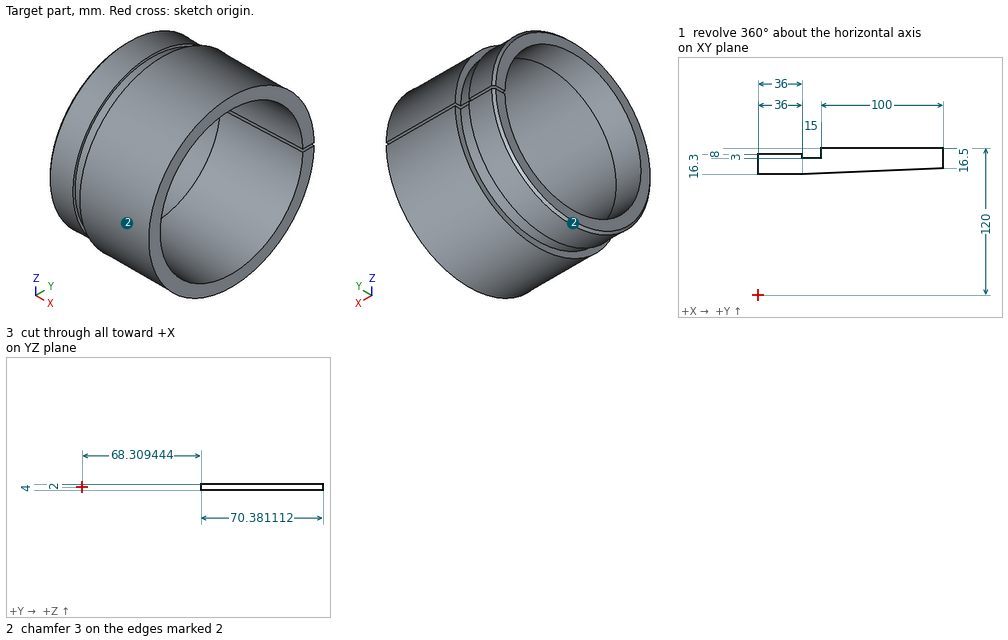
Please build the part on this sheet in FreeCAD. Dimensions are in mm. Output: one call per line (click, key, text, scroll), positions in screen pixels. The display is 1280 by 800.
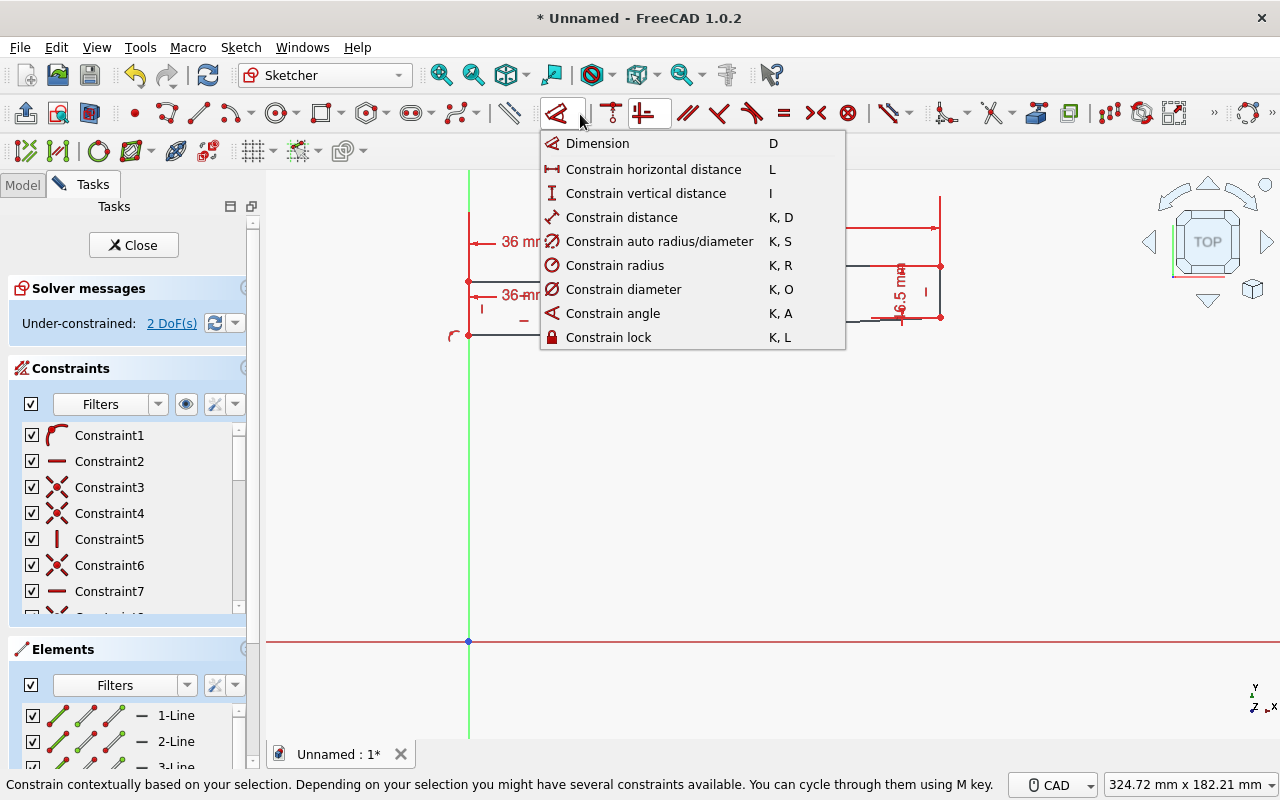
click(693, 193)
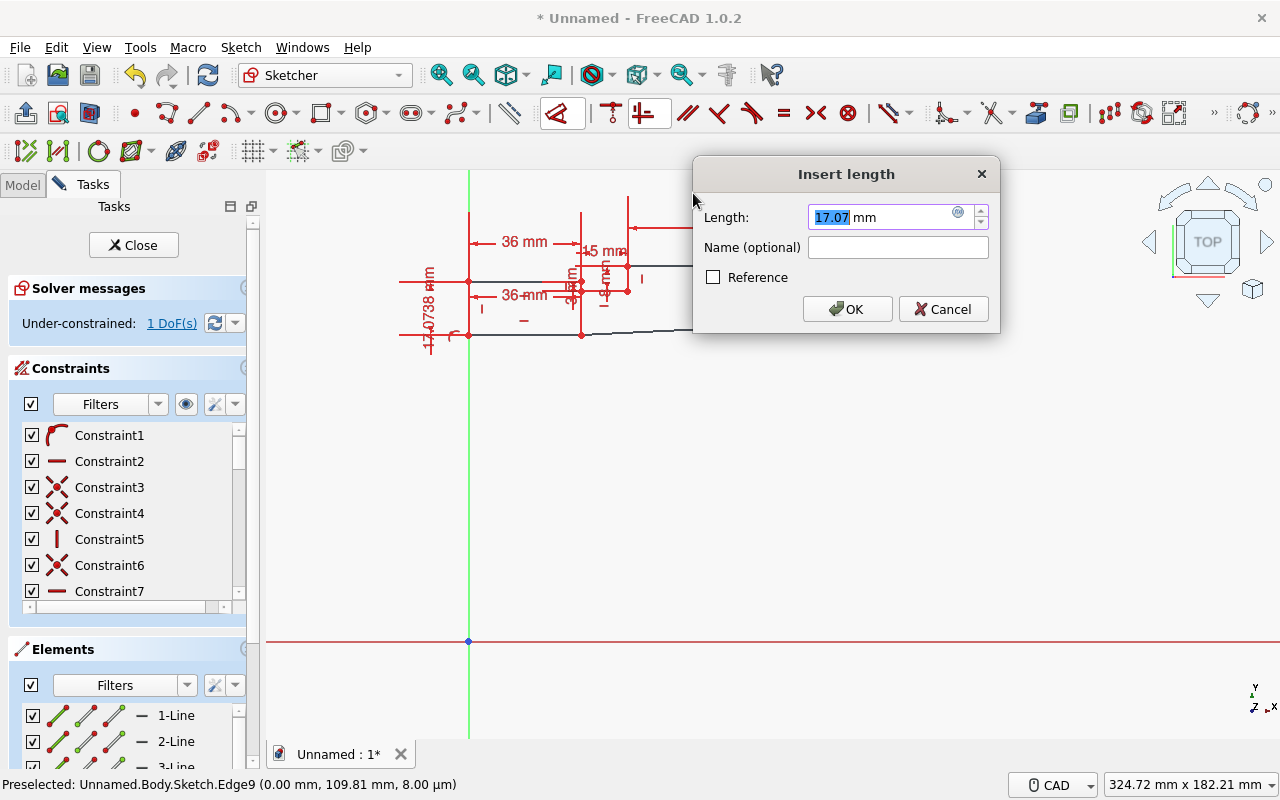
text(16.3)
key(Return)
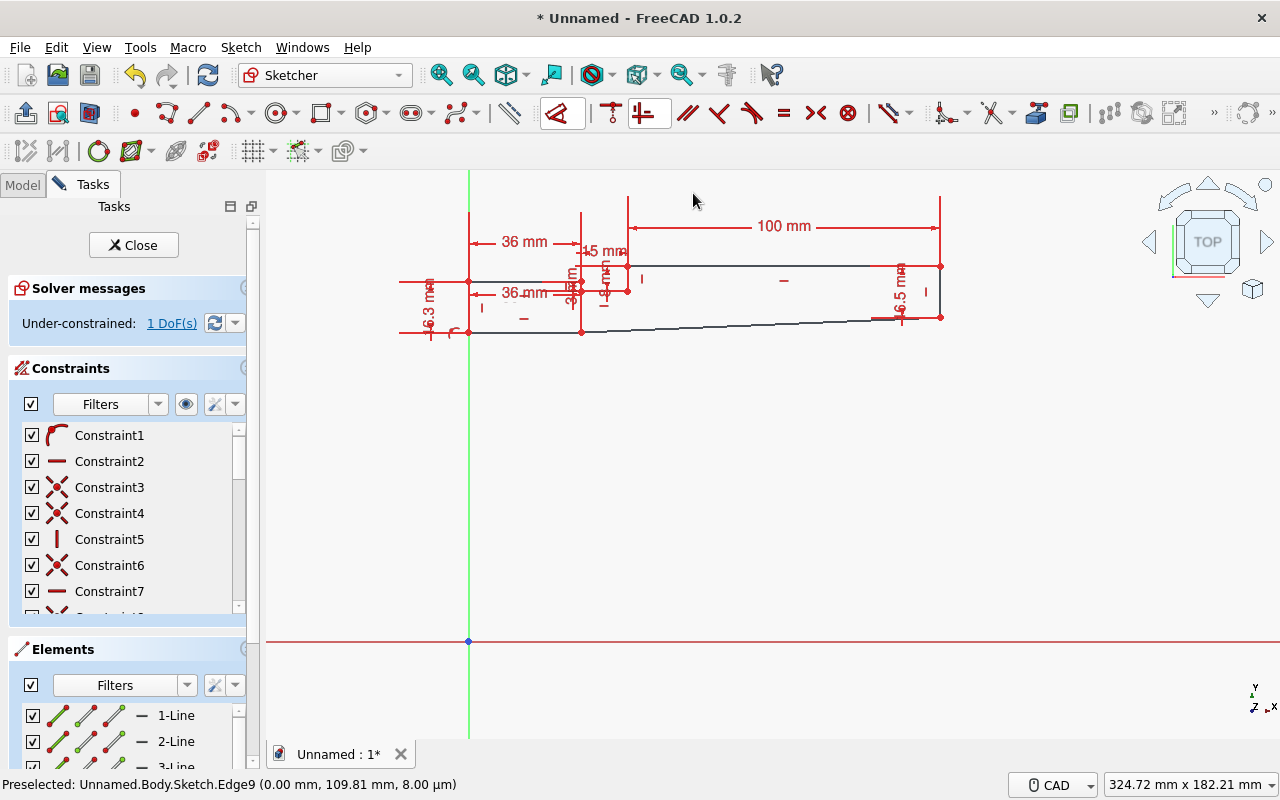
click(940, 266)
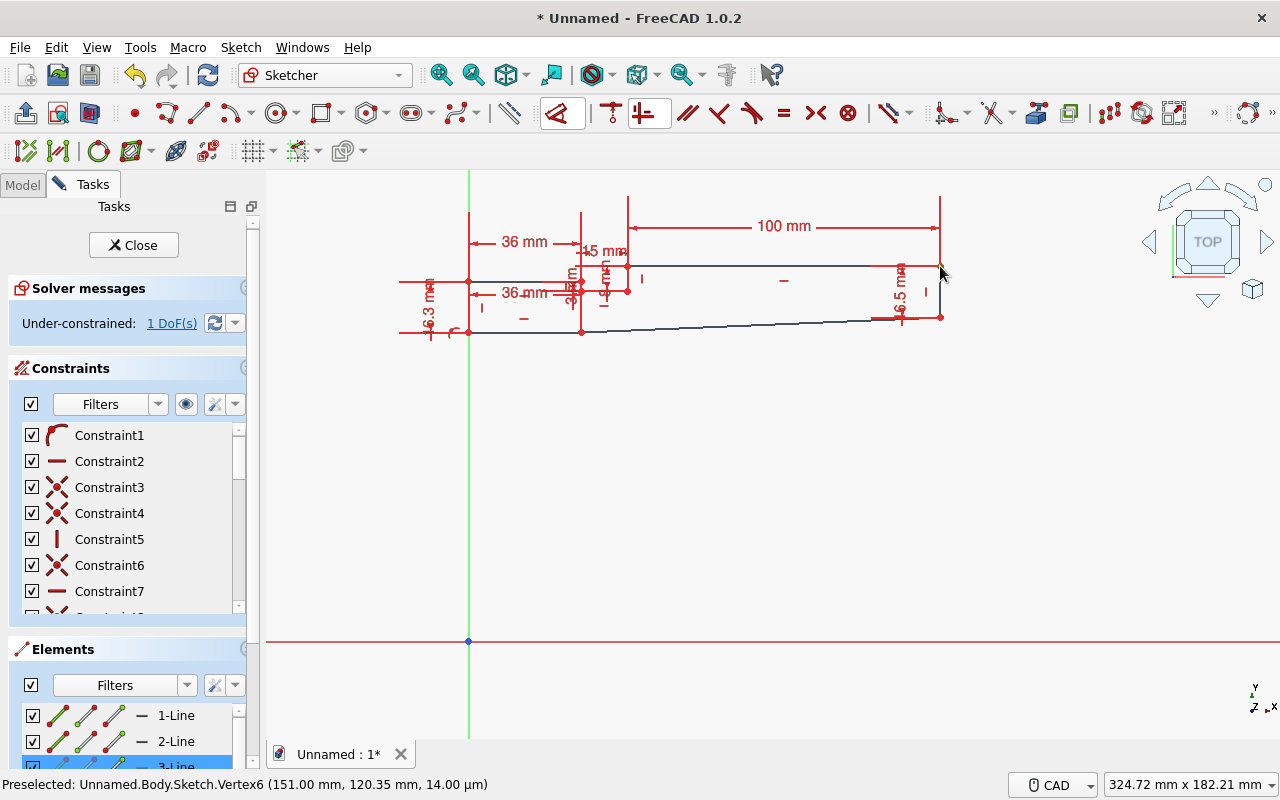
key(i)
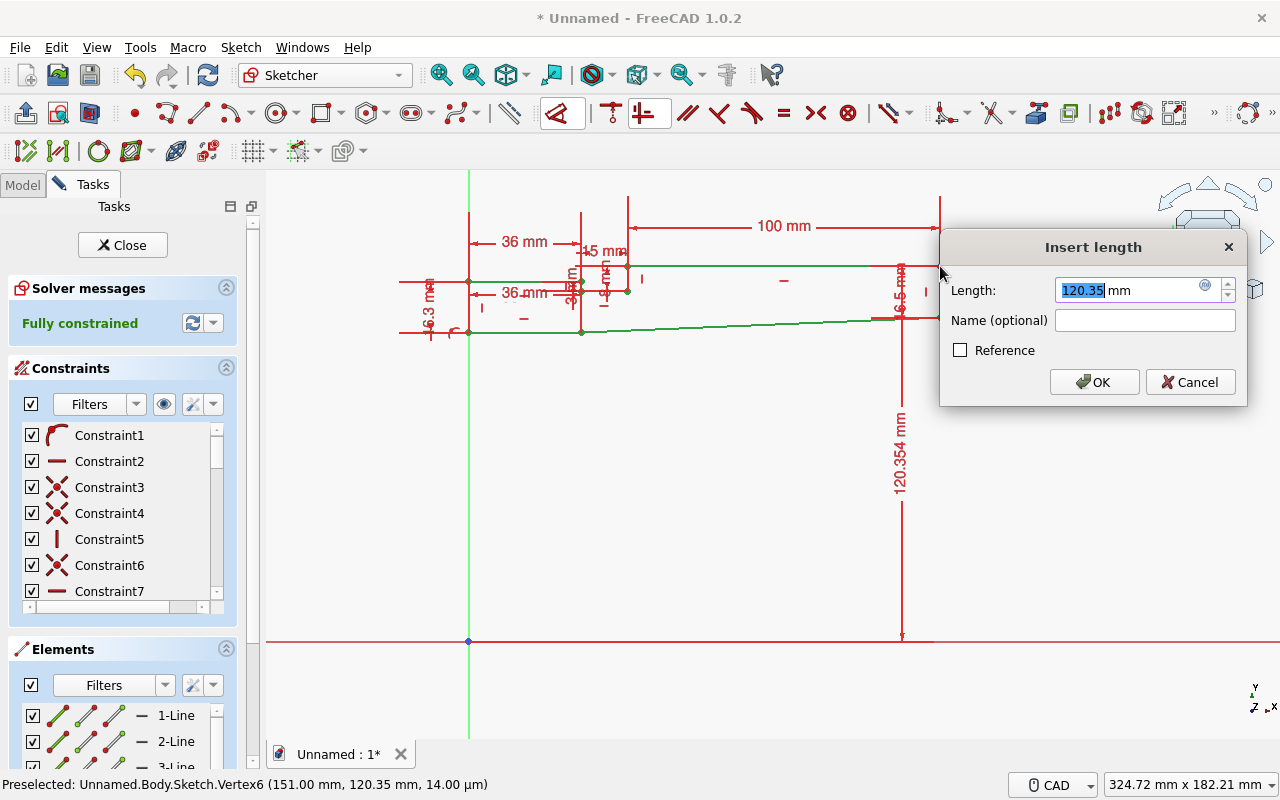
text(120)
key(Return)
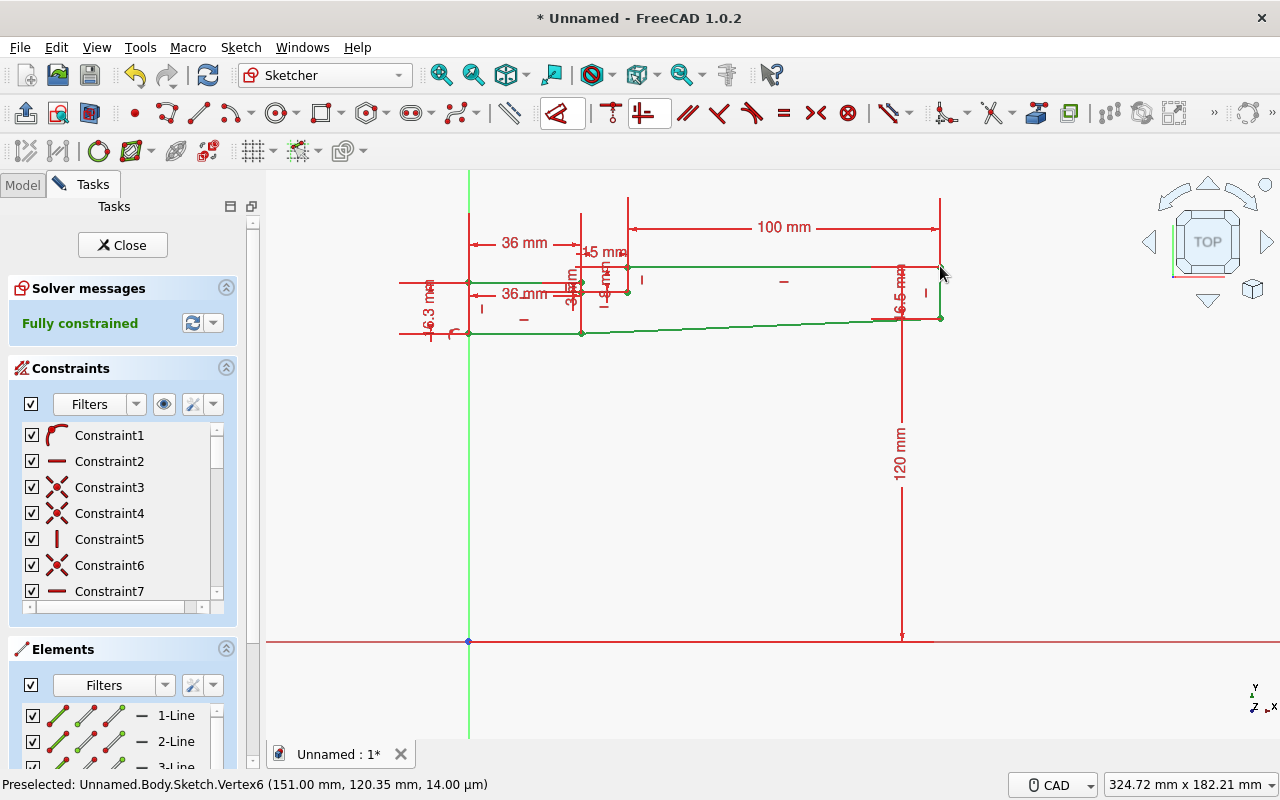
click(123, 245)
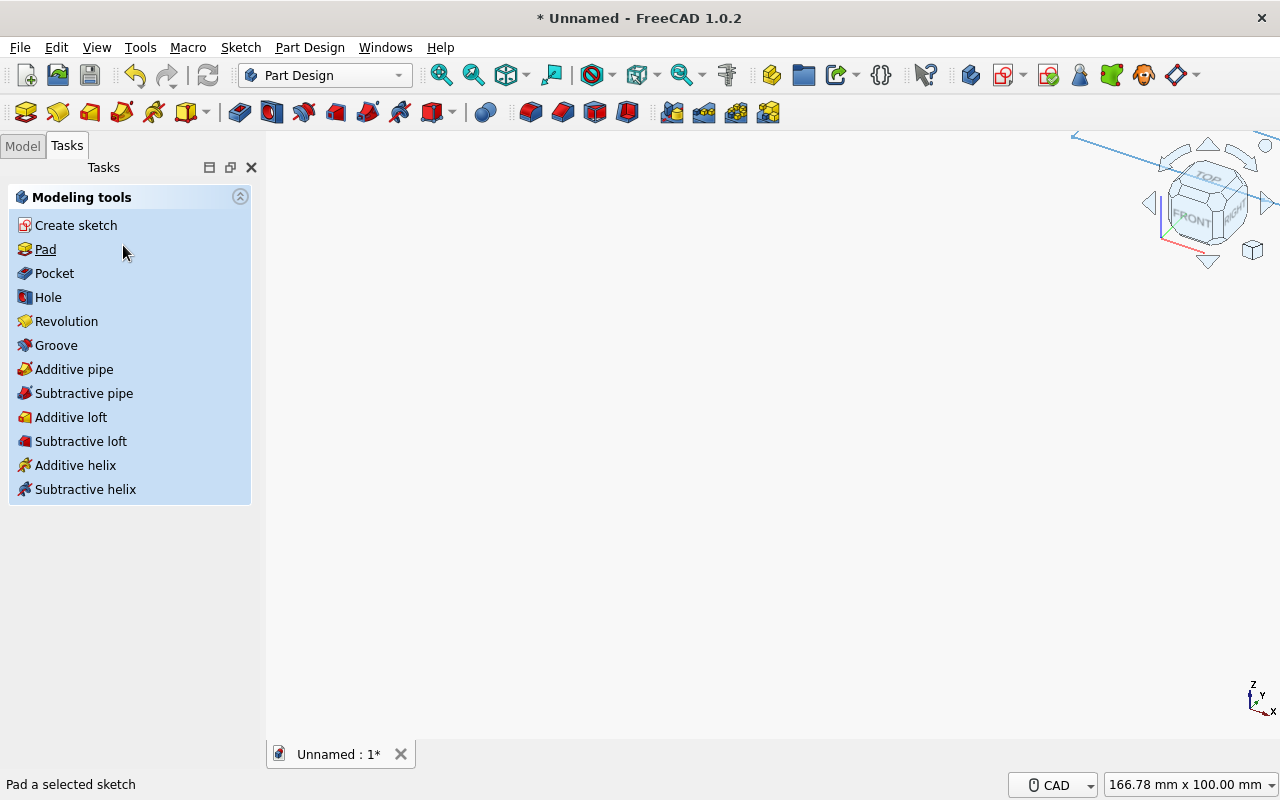
click(58, 112)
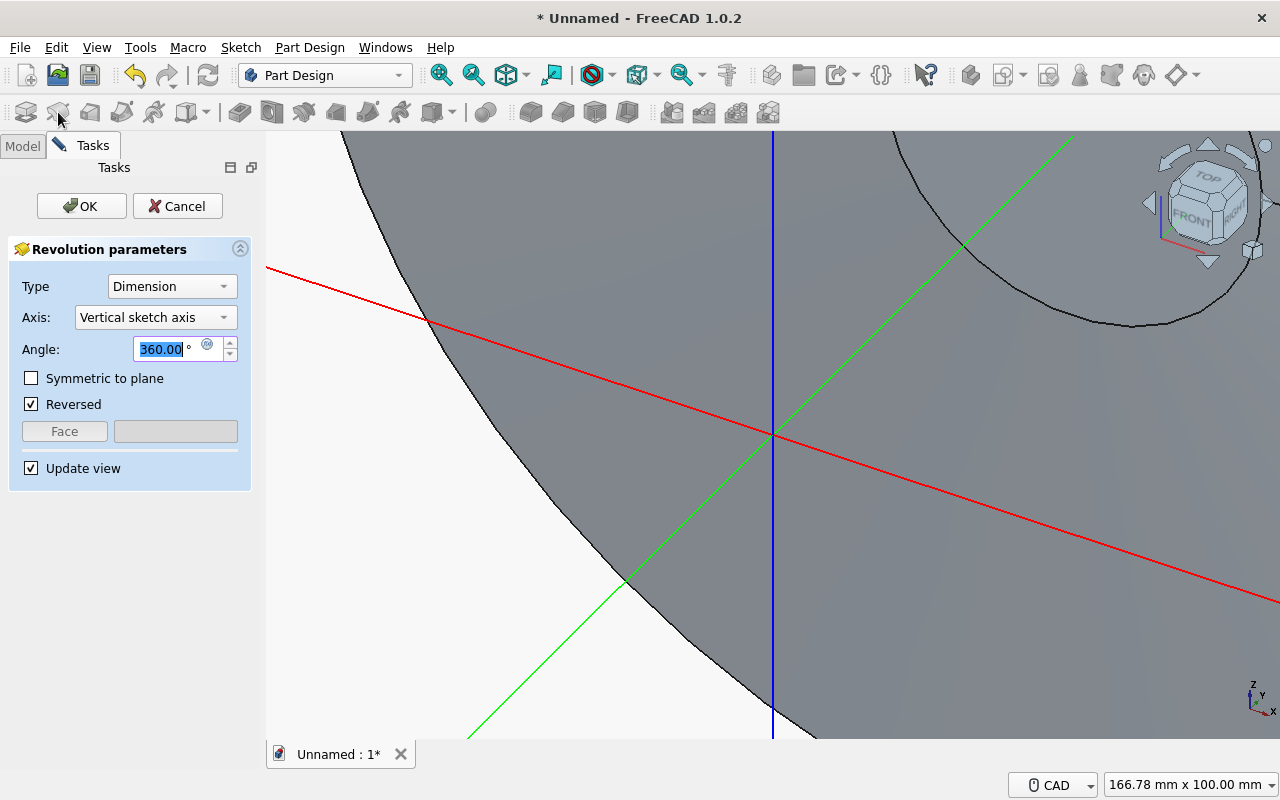
click(156, 318)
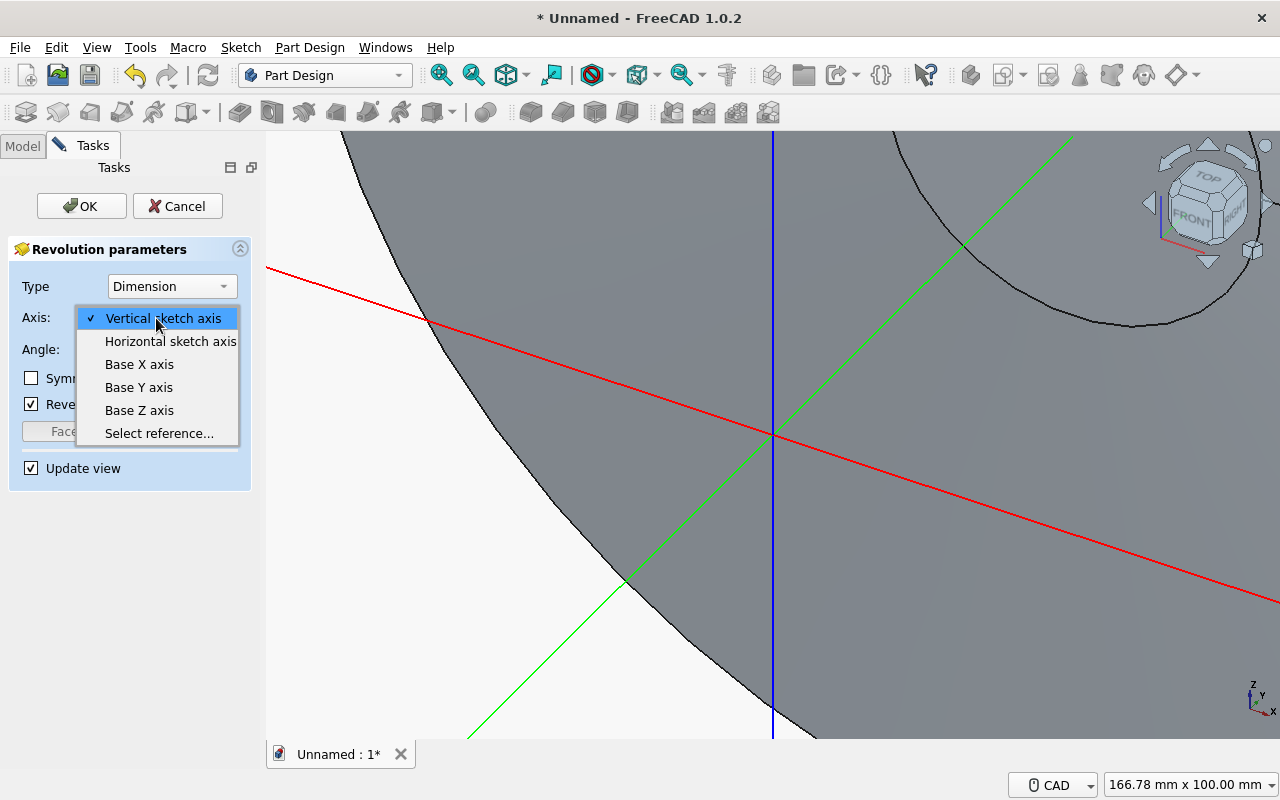
click(156, 342)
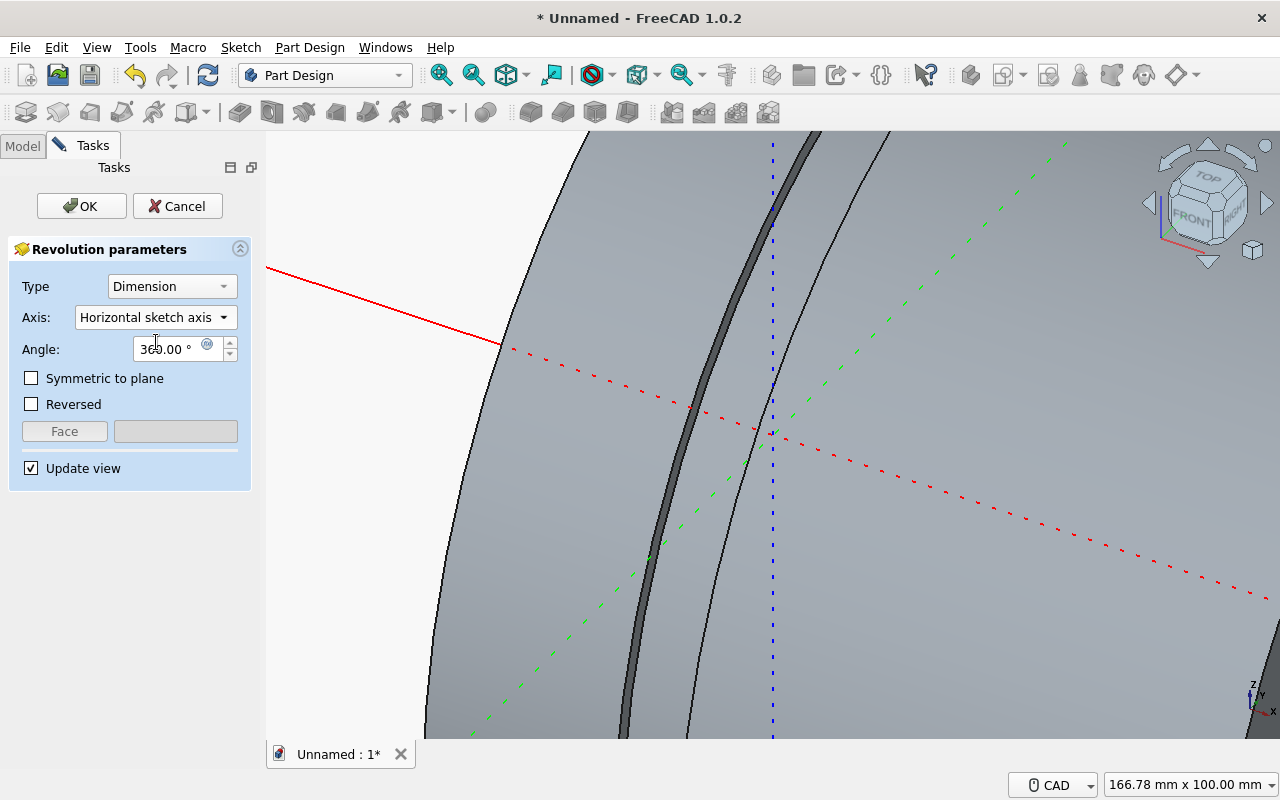
click(82, 206)